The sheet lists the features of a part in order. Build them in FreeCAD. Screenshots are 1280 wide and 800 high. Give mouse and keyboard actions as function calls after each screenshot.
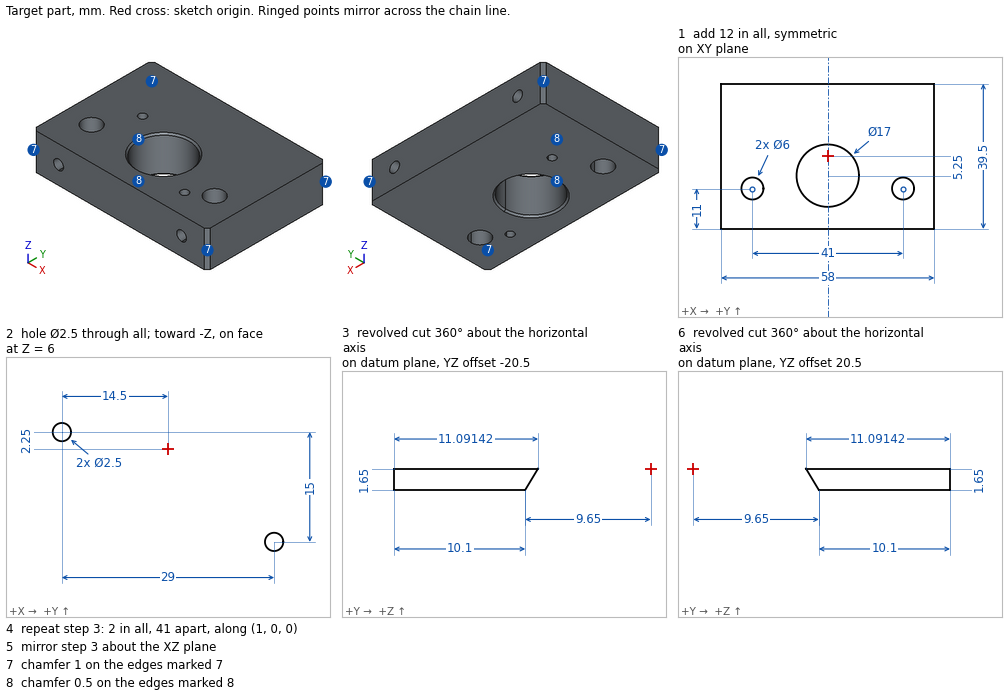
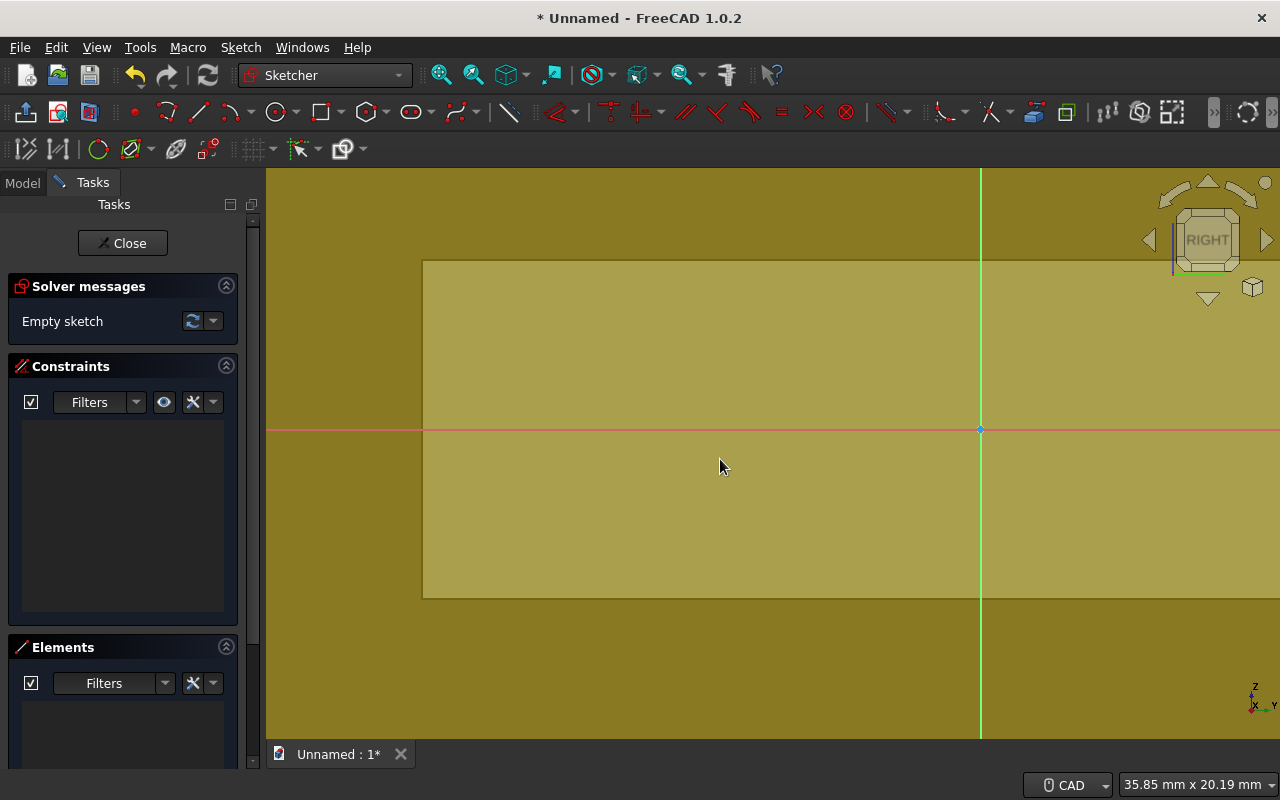
key(g)
key(m)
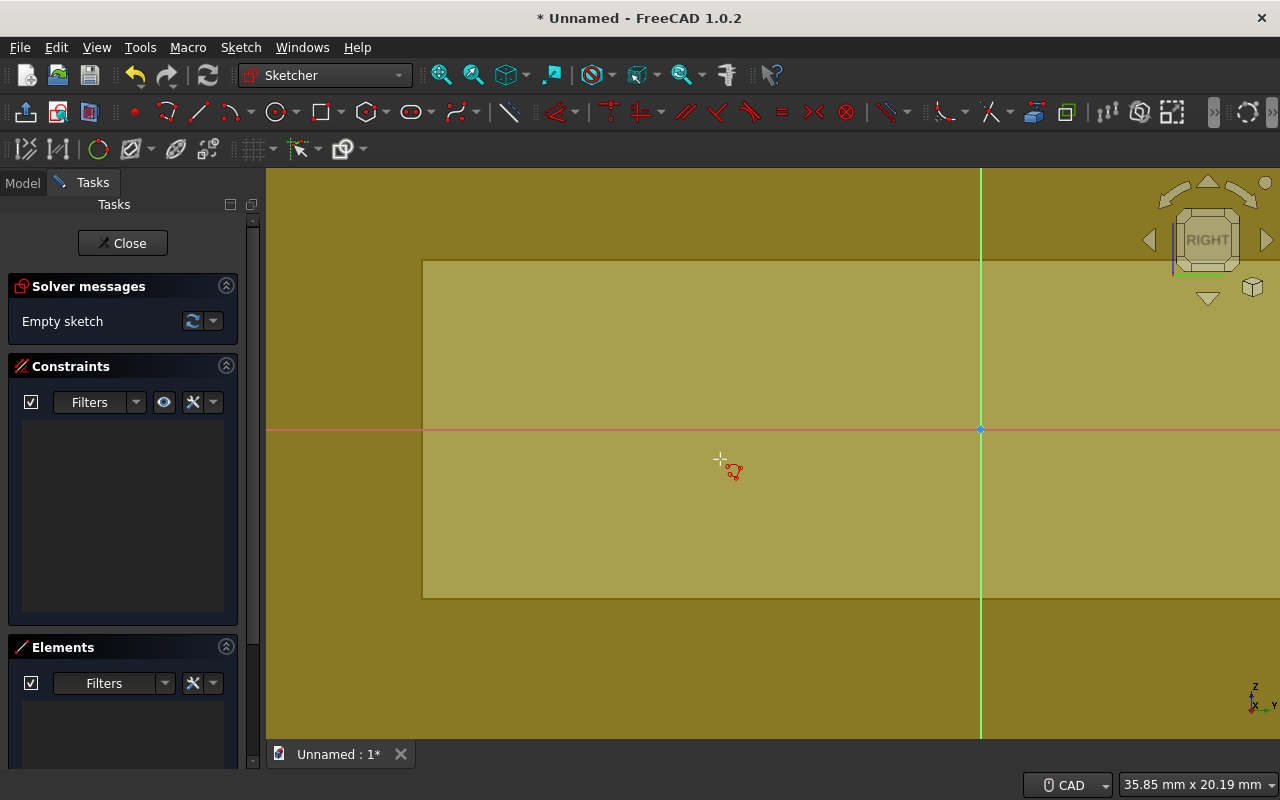
click(736, 430)
click(422, 439)
click(422, 476)
click(708, 476)
click(736, 430)
key(Escape)
key(Escape)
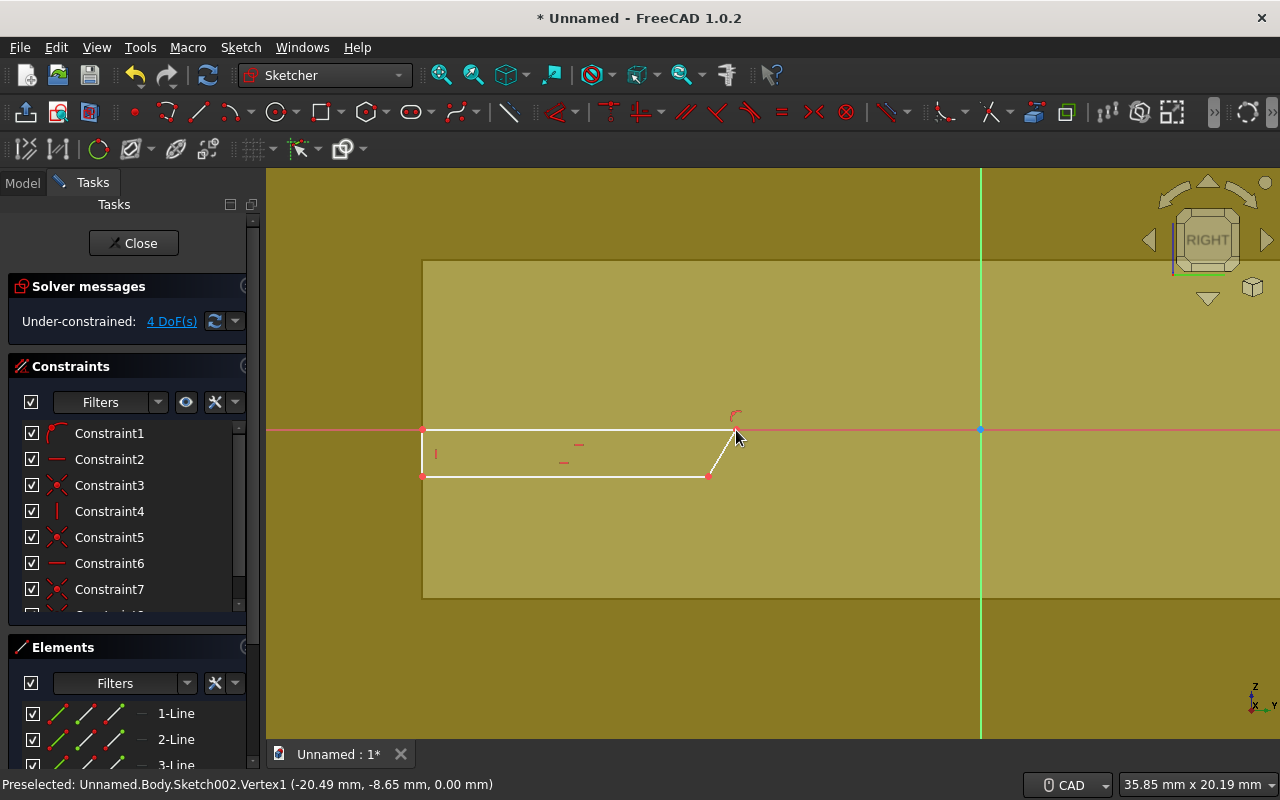
click(556, 112)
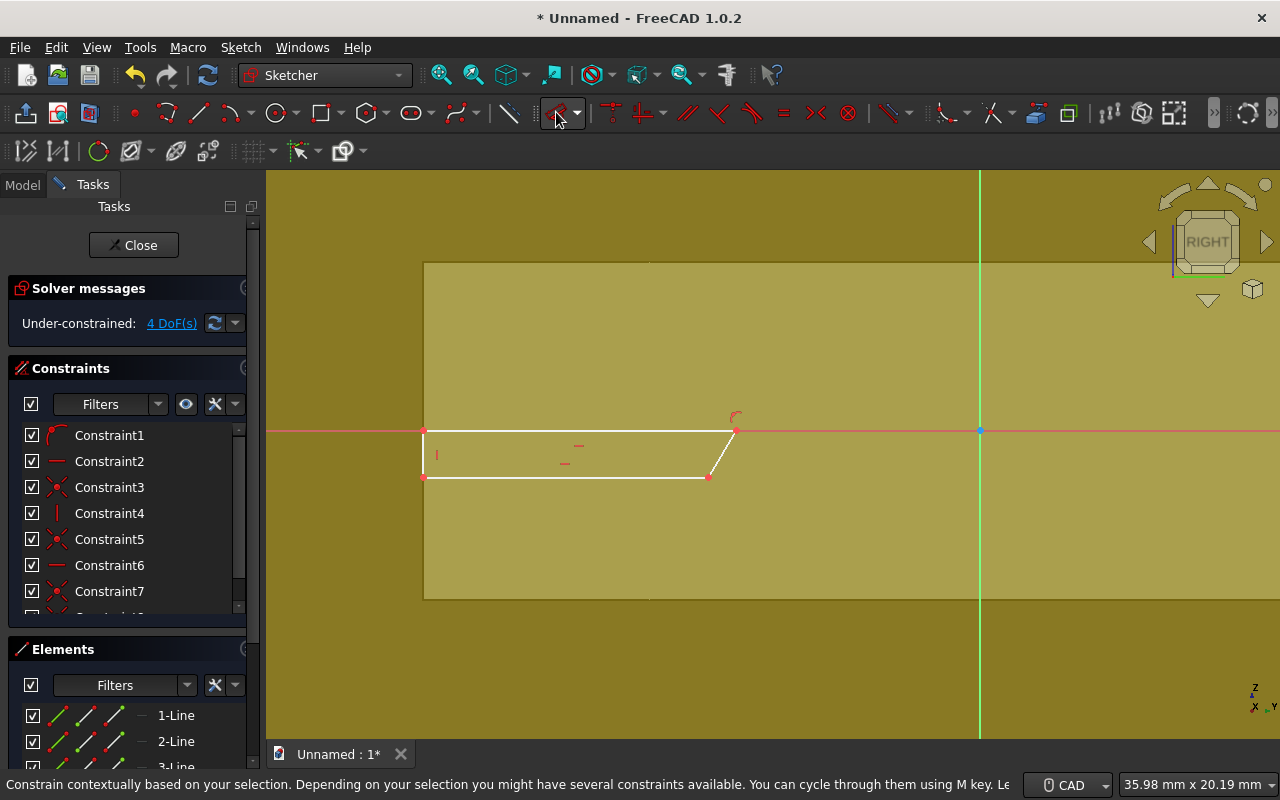
click(423, 445)
click(389, 454)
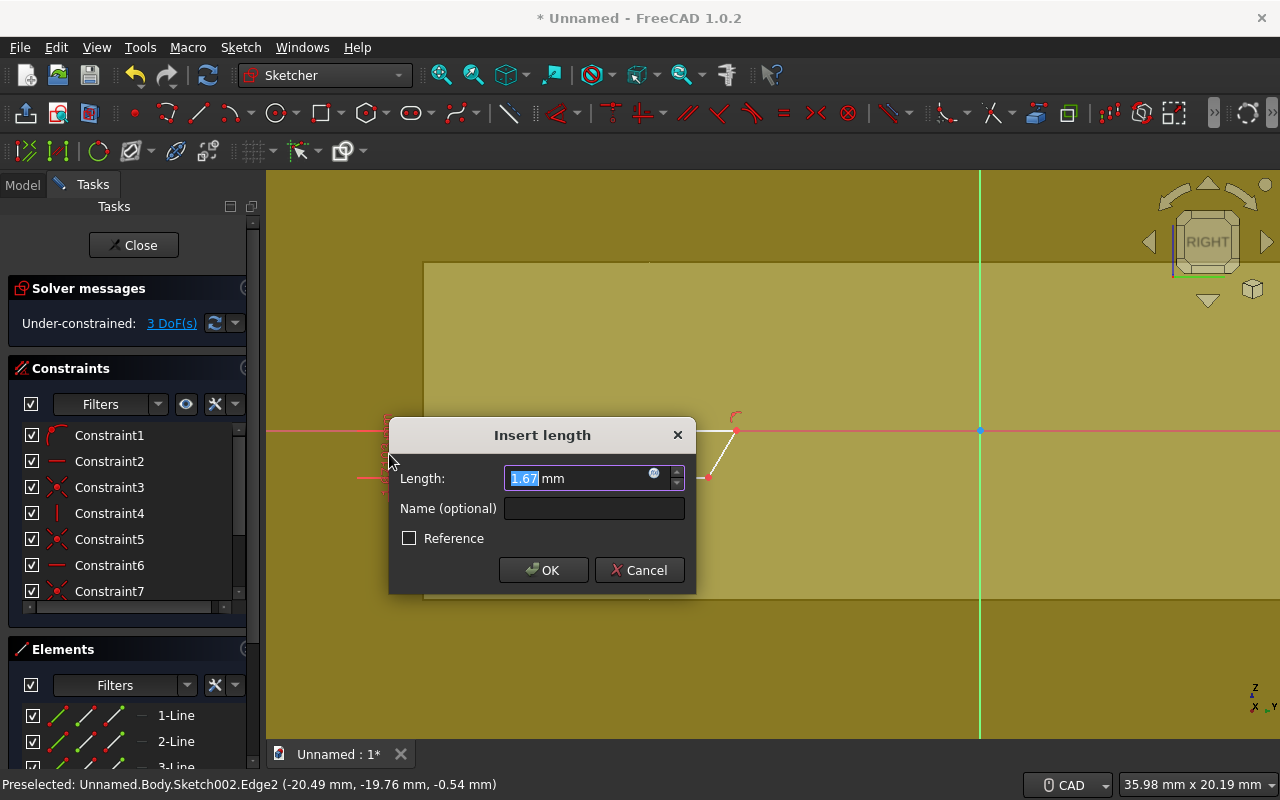
text(1.65)
key(Return)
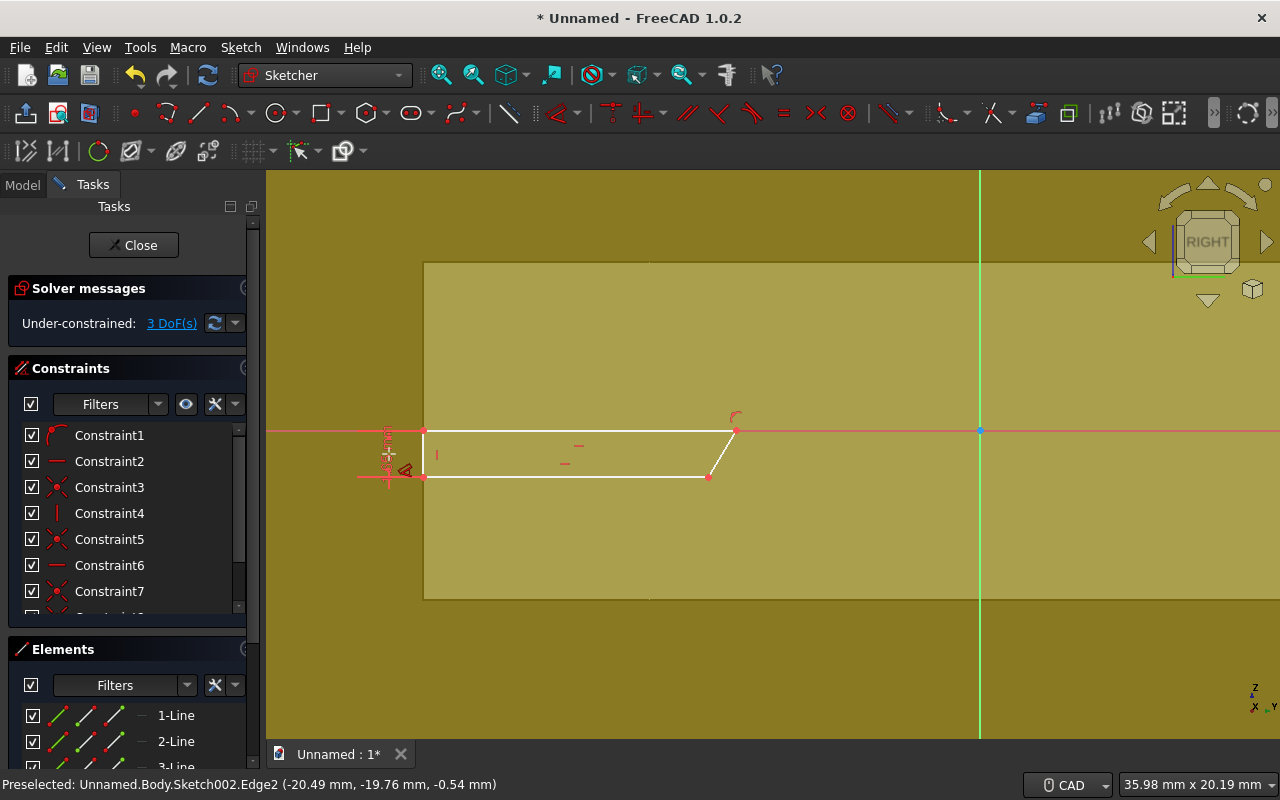
click(509, 477)
click(566, 511)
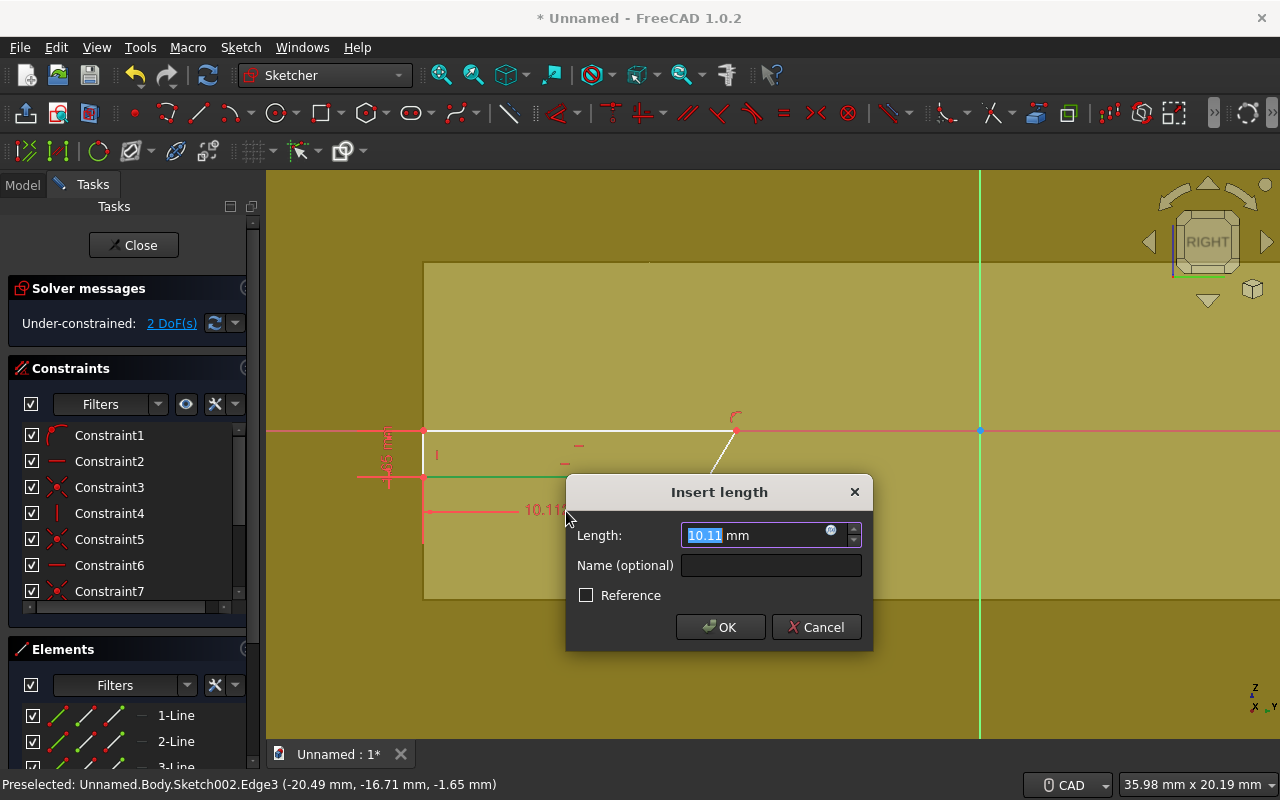
text(10.1)
key(Return)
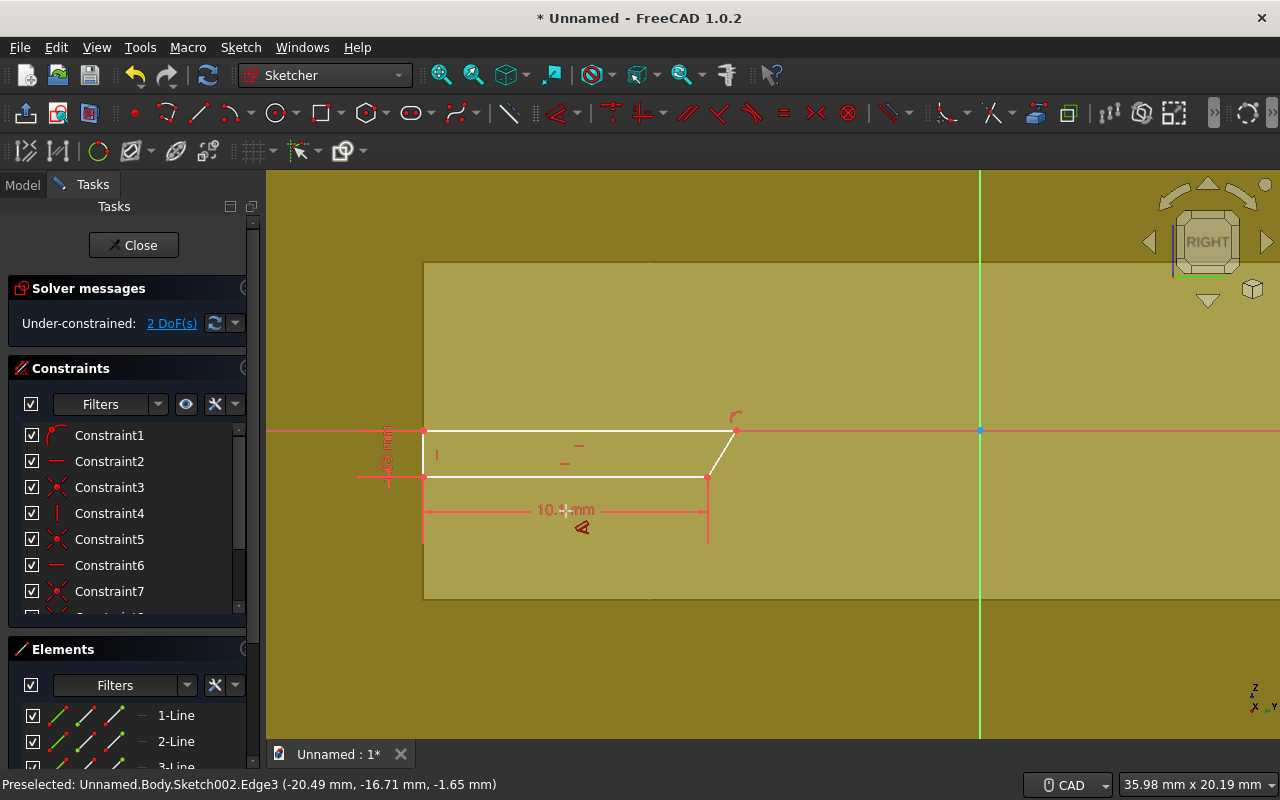
click(708, 477)
click(844, 511)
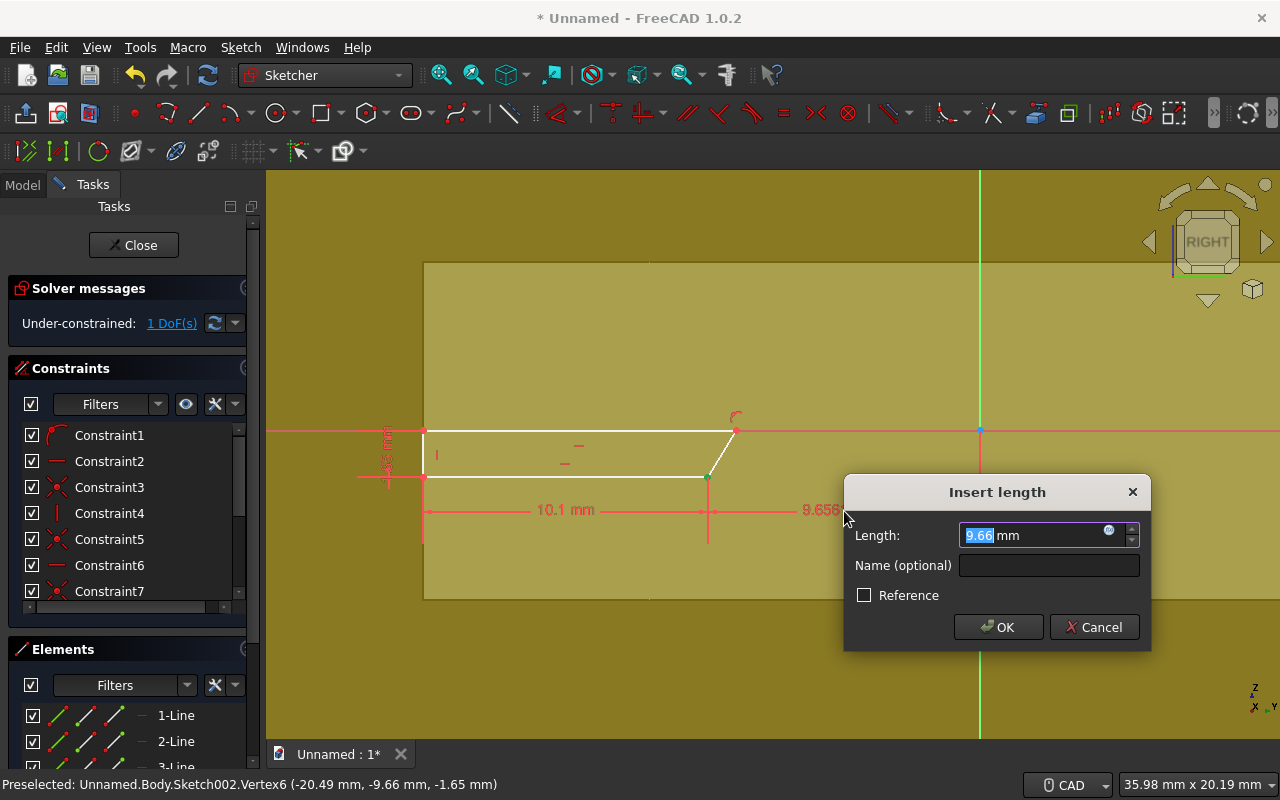
text(9.65)
key(Return)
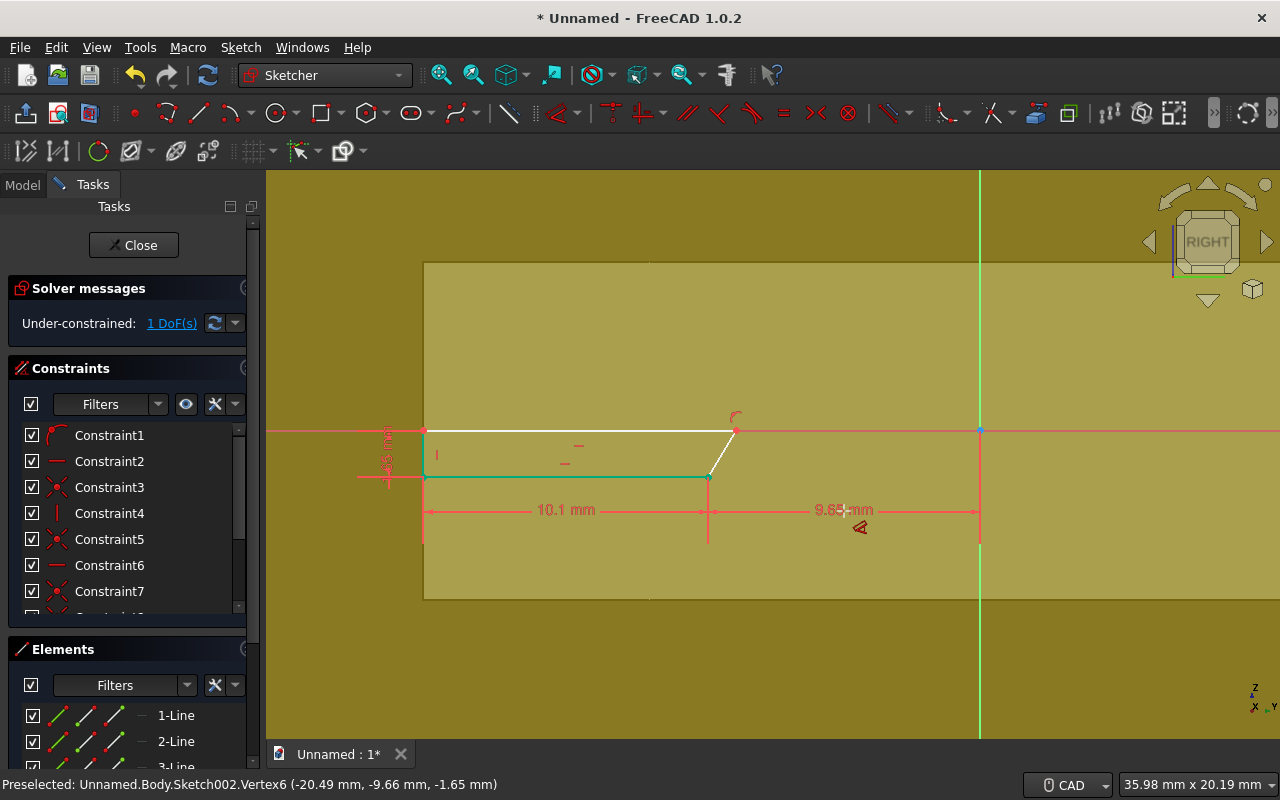
click(642, 431)
click(580, 397)